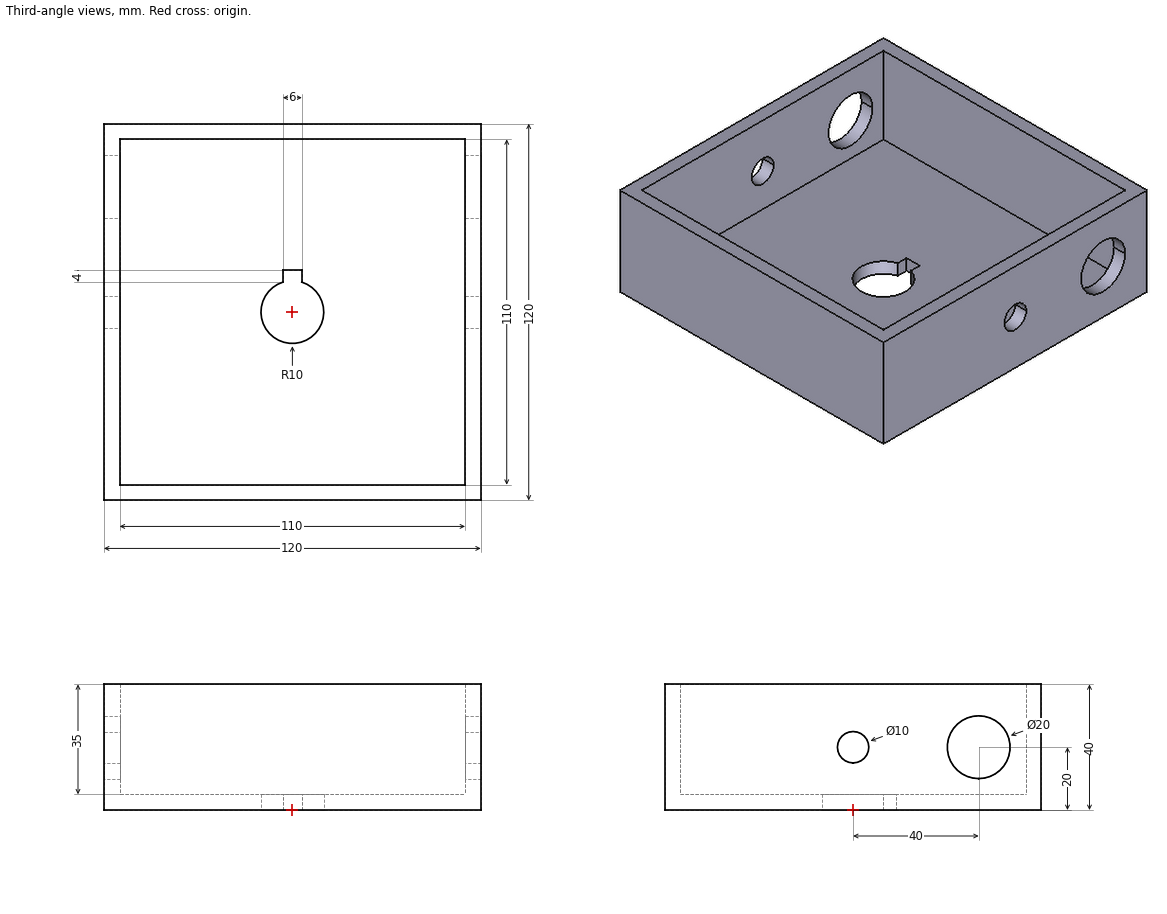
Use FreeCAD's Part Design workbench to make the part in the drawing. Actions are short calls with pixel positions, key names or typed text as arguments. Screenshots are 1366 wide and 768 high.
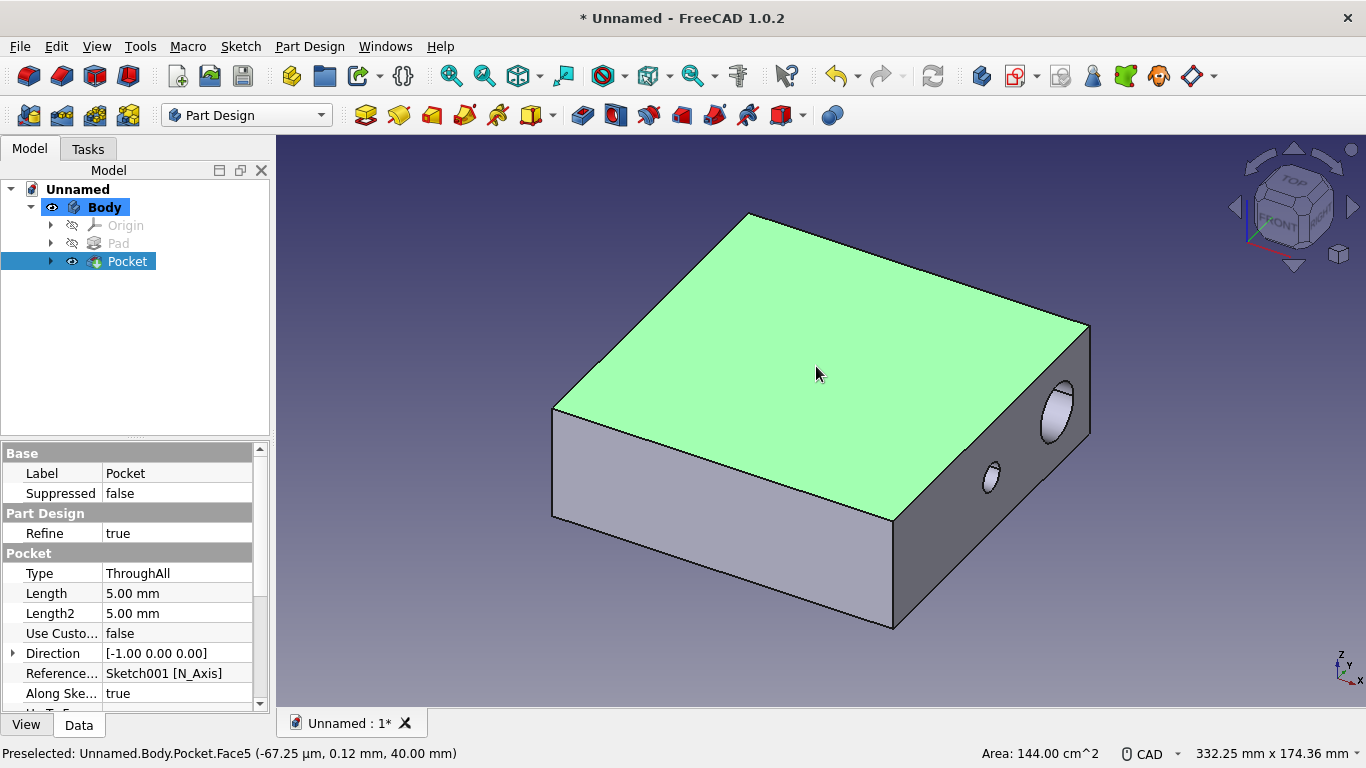
click(1014, 76)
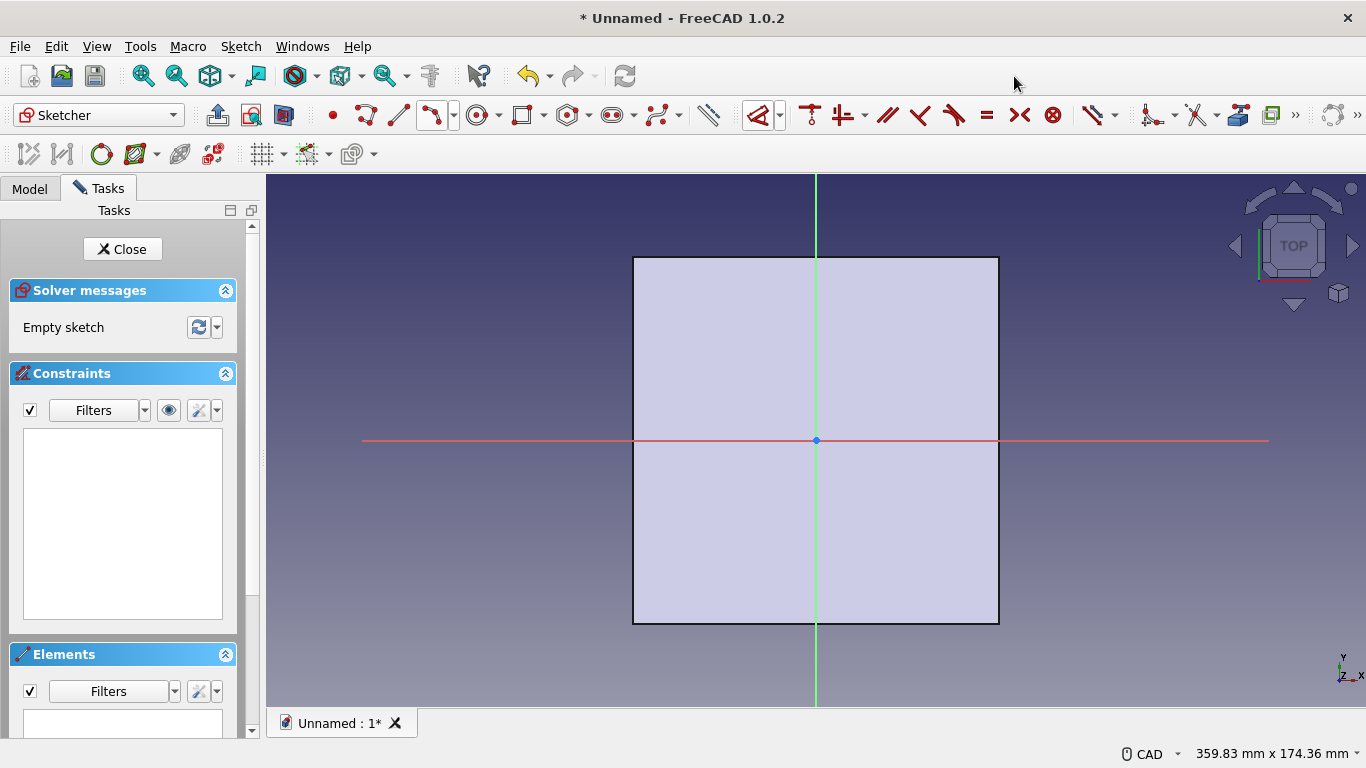
key(g)
key(v)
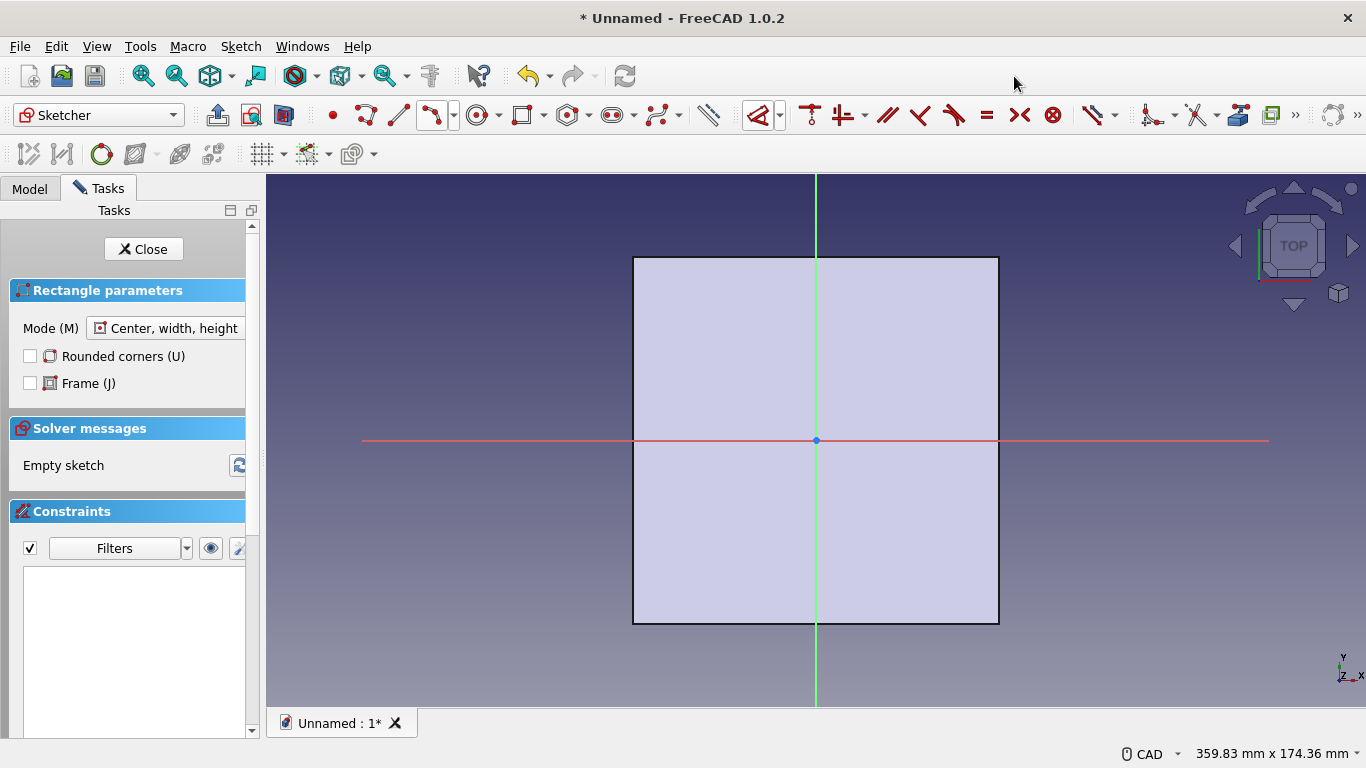
click(816, 441)
move(984, 272)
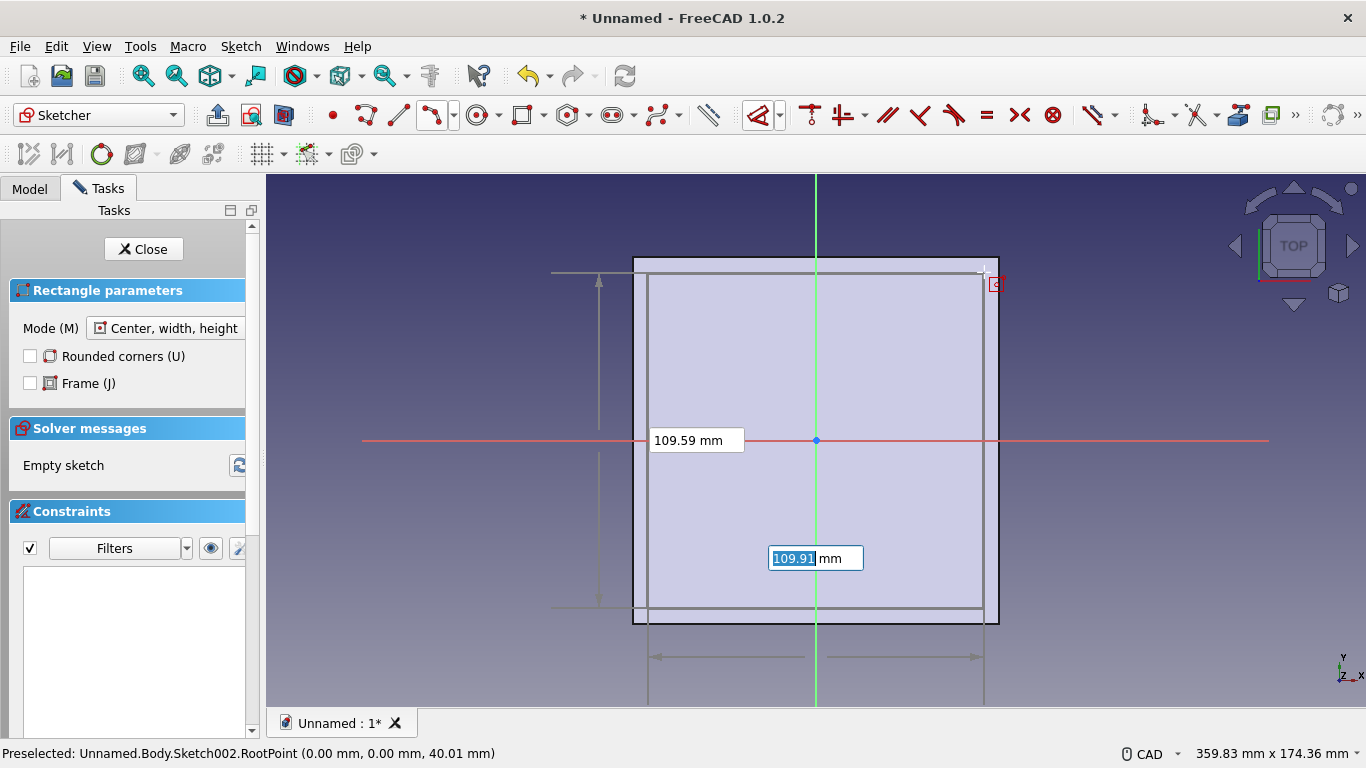
text(110)
key(Tab)
text(110)
key(Return)
key(Escape)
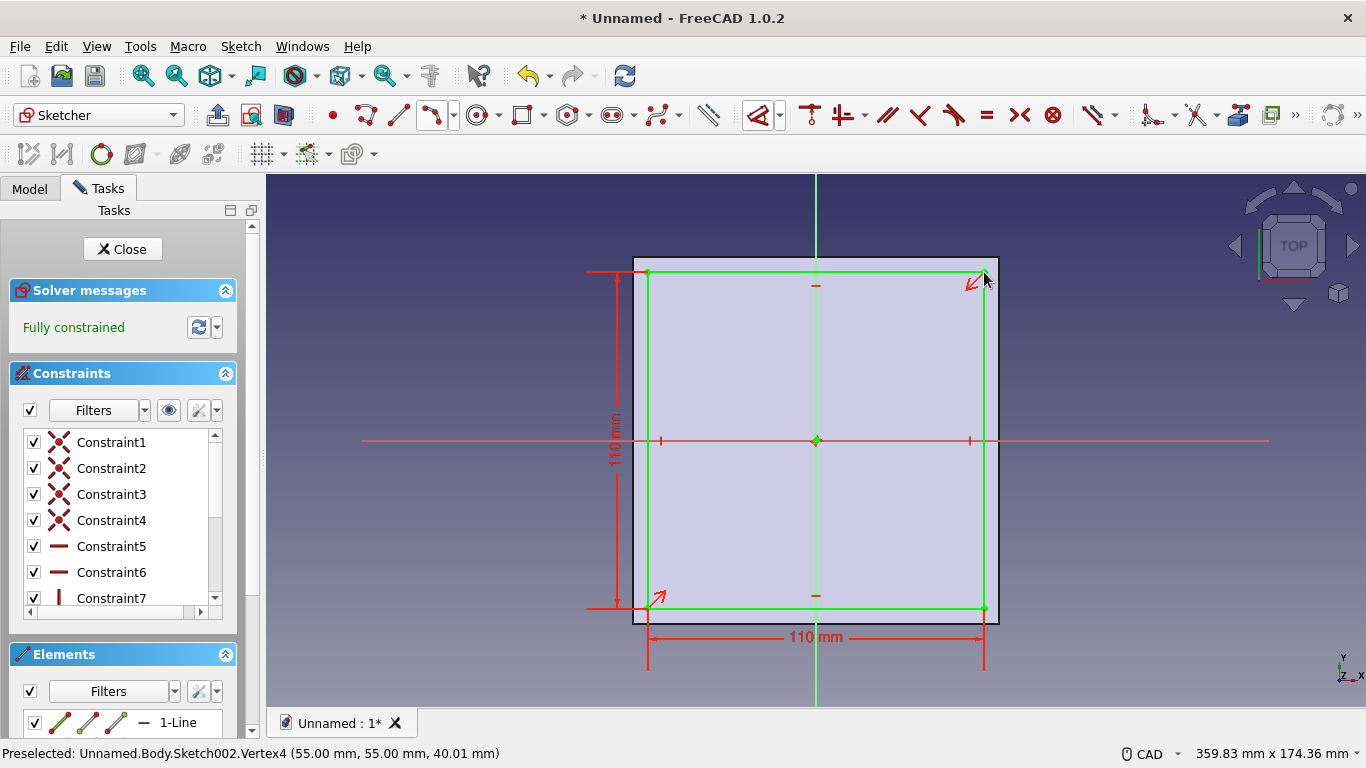
click(123, 249)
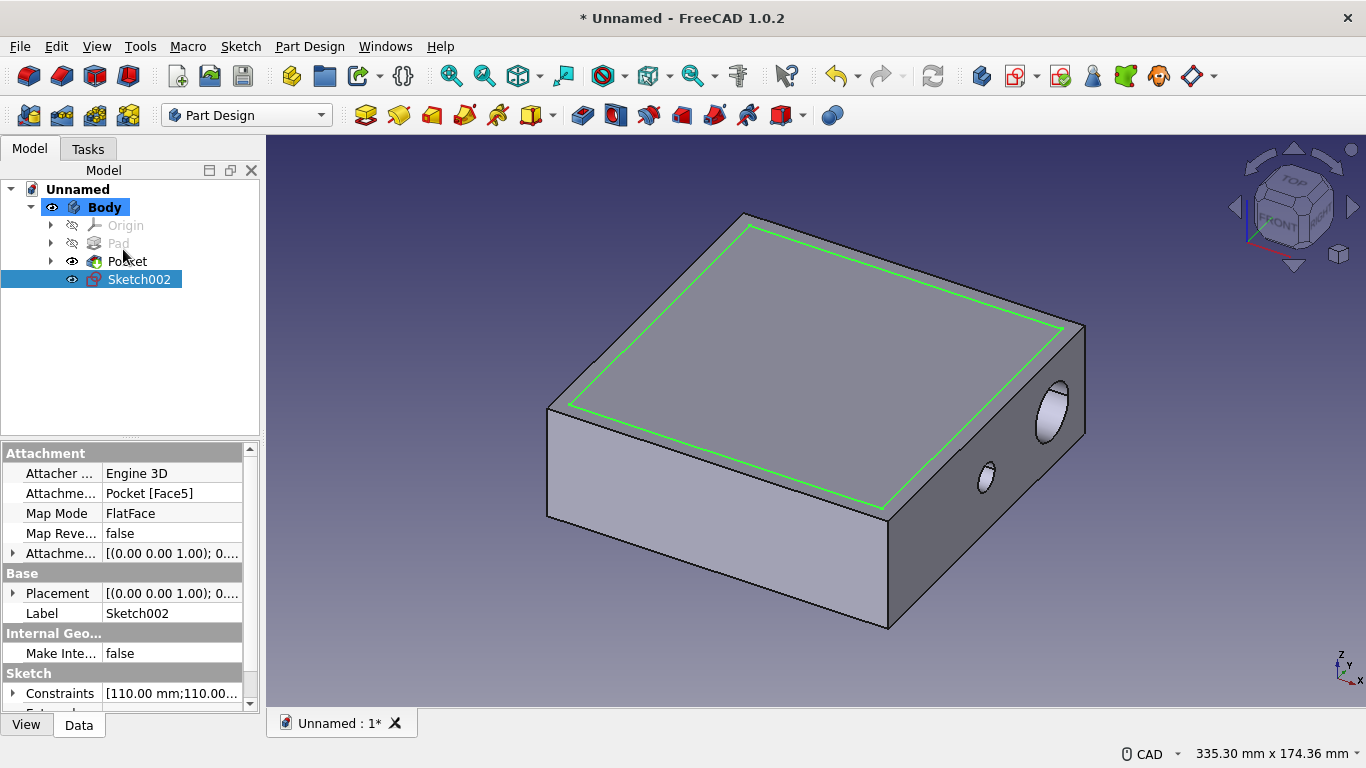
click(583, 116)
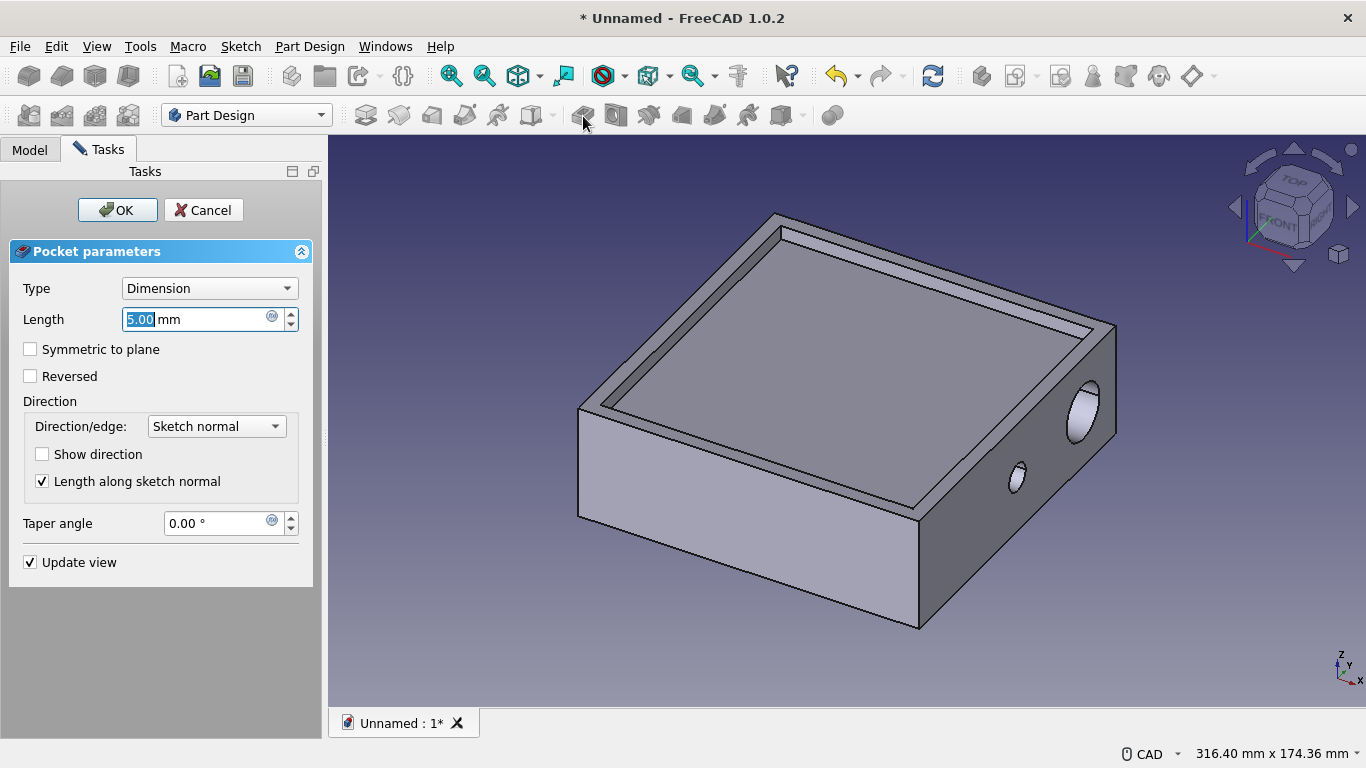
text(35)
key(Tab)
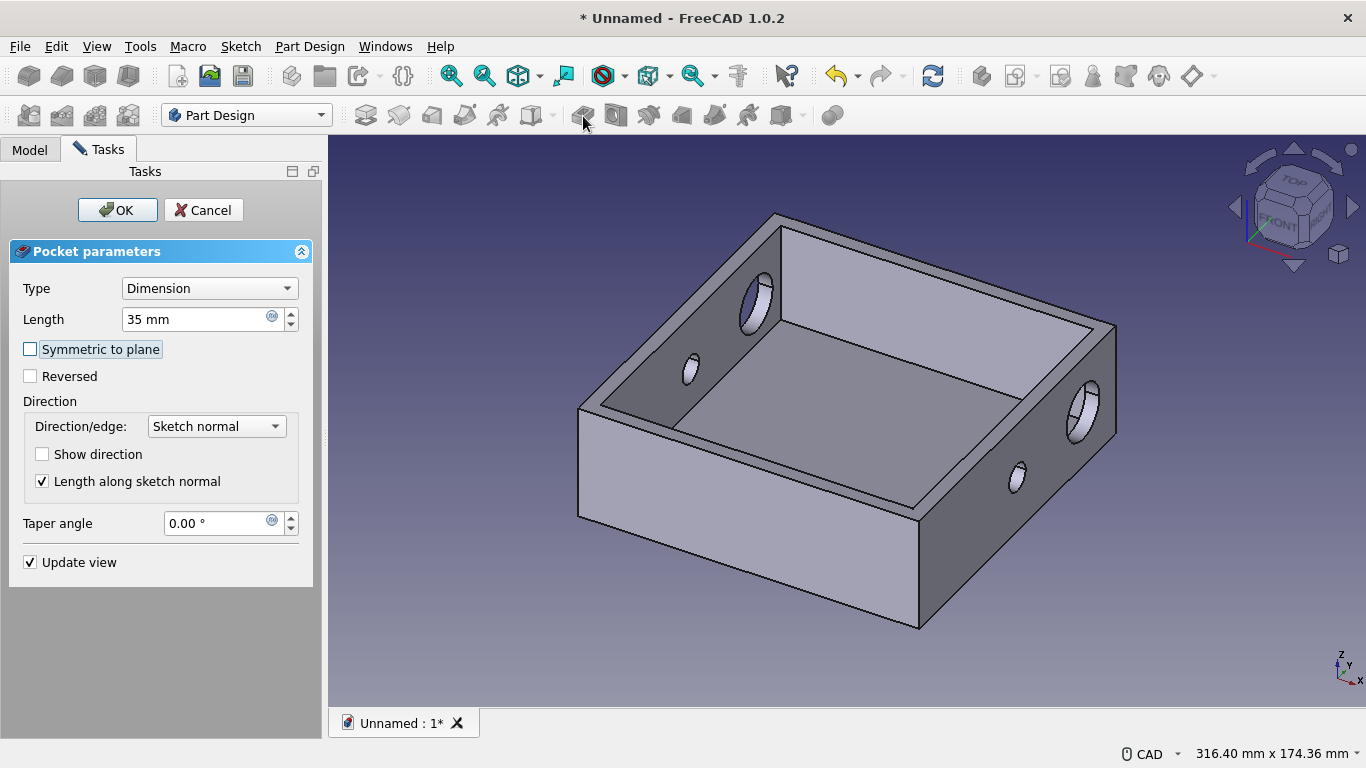
click(118, 210)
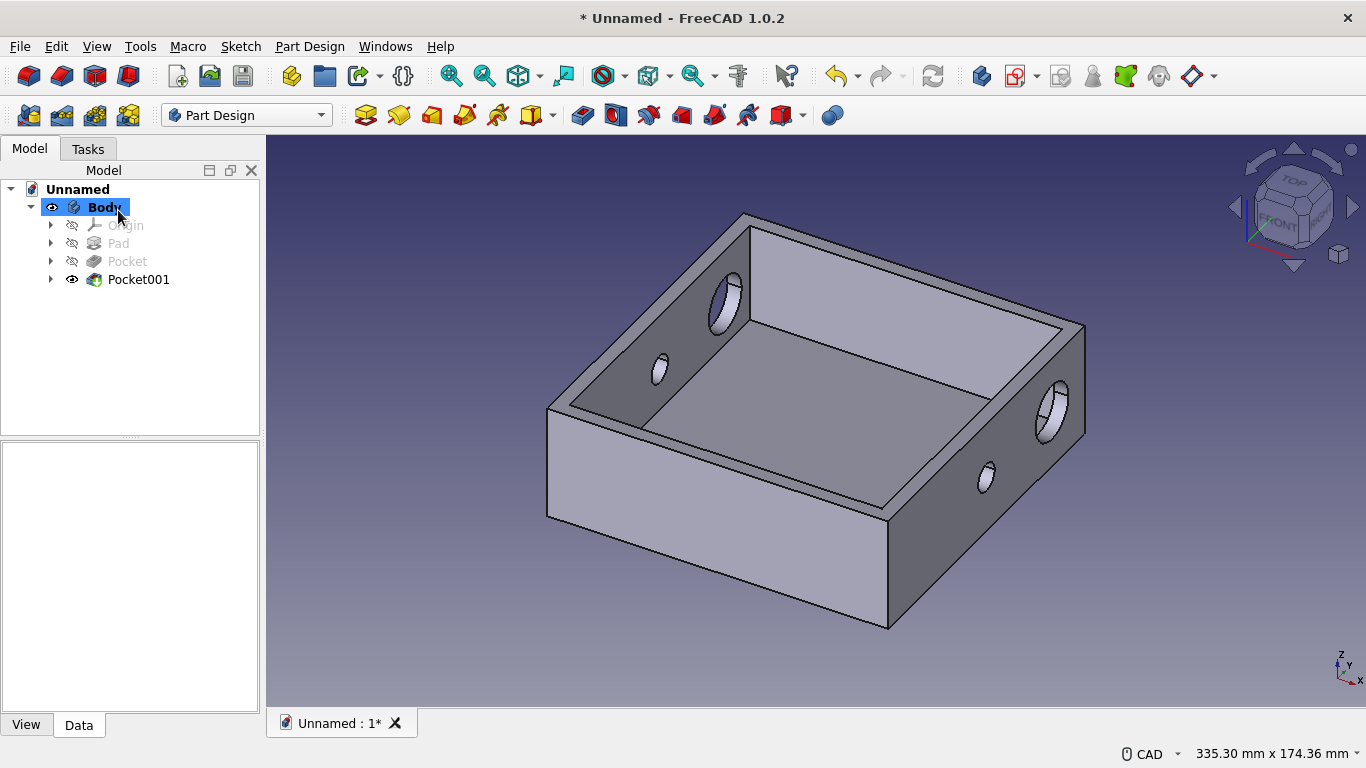
click(1014, 76)